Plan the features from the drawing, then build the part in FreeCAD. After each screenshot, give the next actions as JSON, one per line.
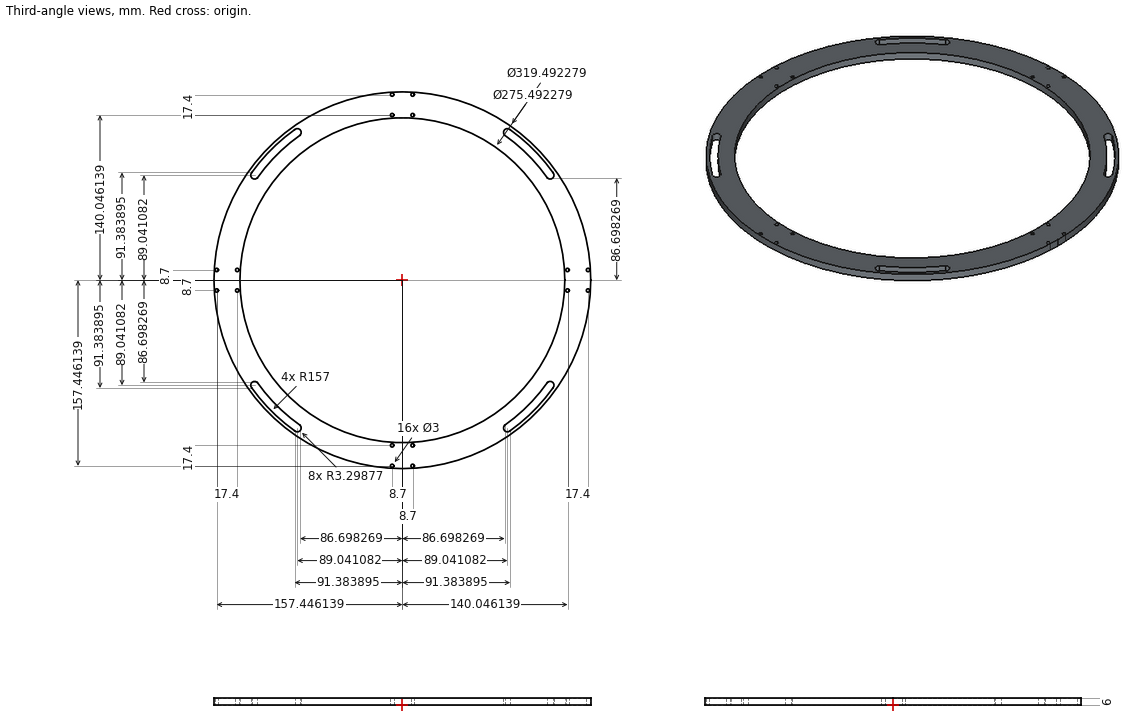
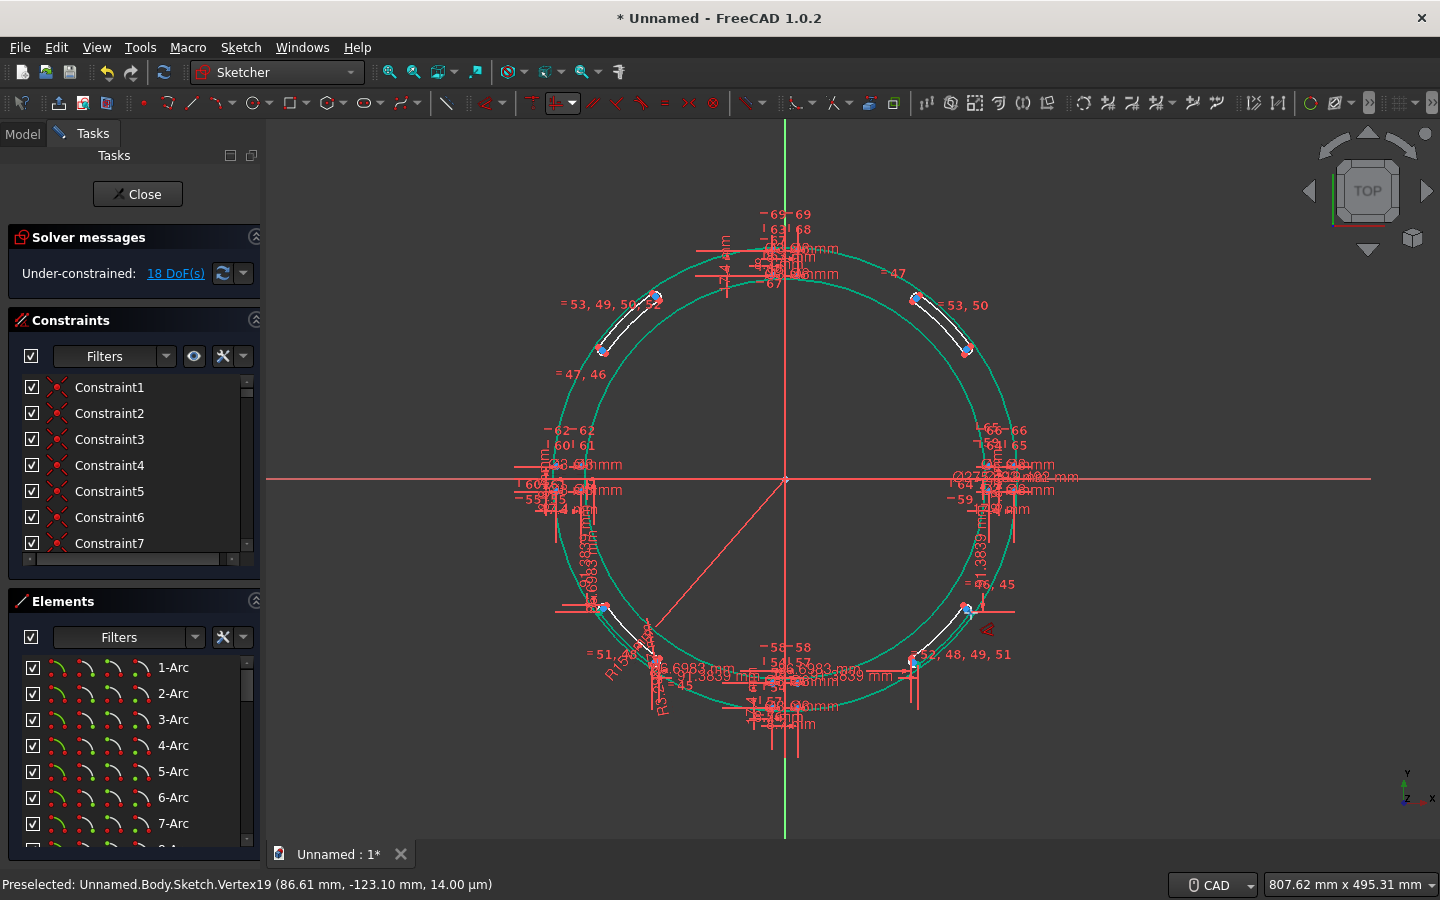
{"action": "scroll", "coordinate": [599, 347], "scroll_direction": "up", "scroll_amount": 5}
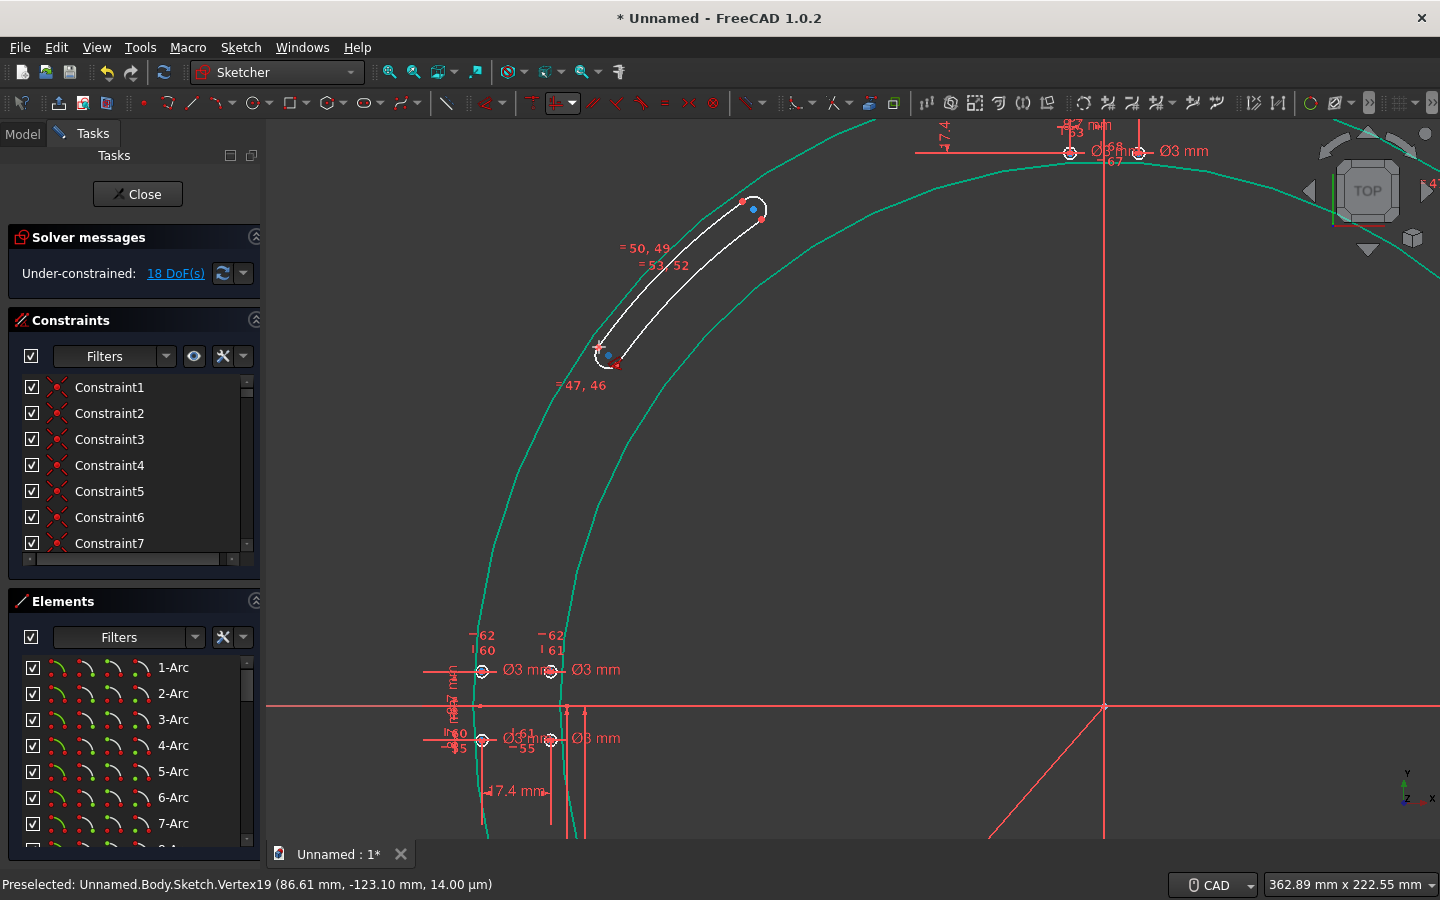
{"action": "left_click", "coordinate": [598, 348]}
{"action": "left_click", "coordinate": [564, 527]}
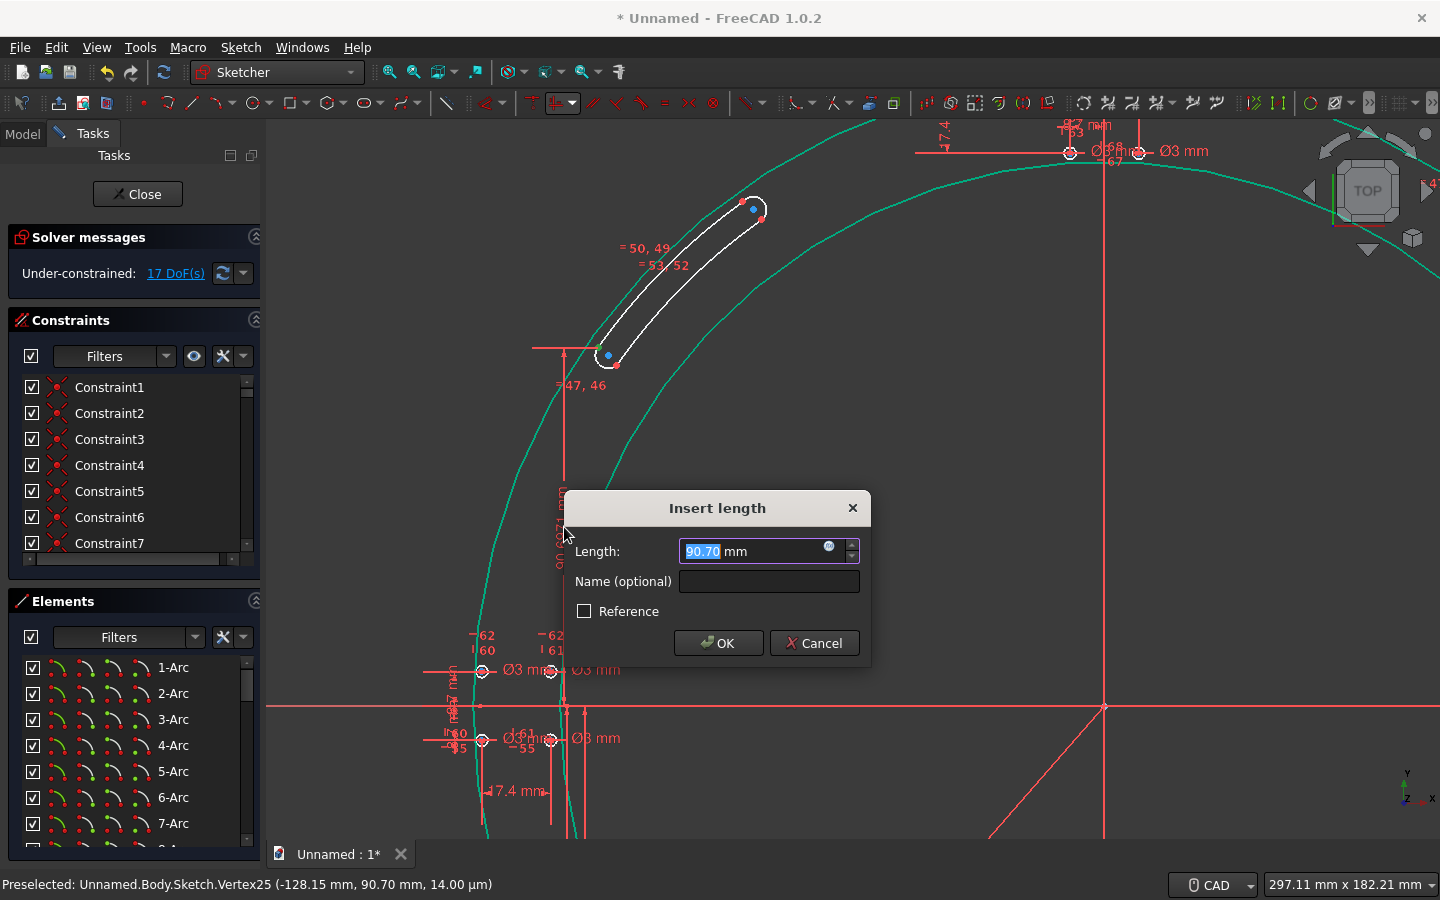
{"action": "type", "text": "91.383895"}
{"action": "key", "text": "Return"}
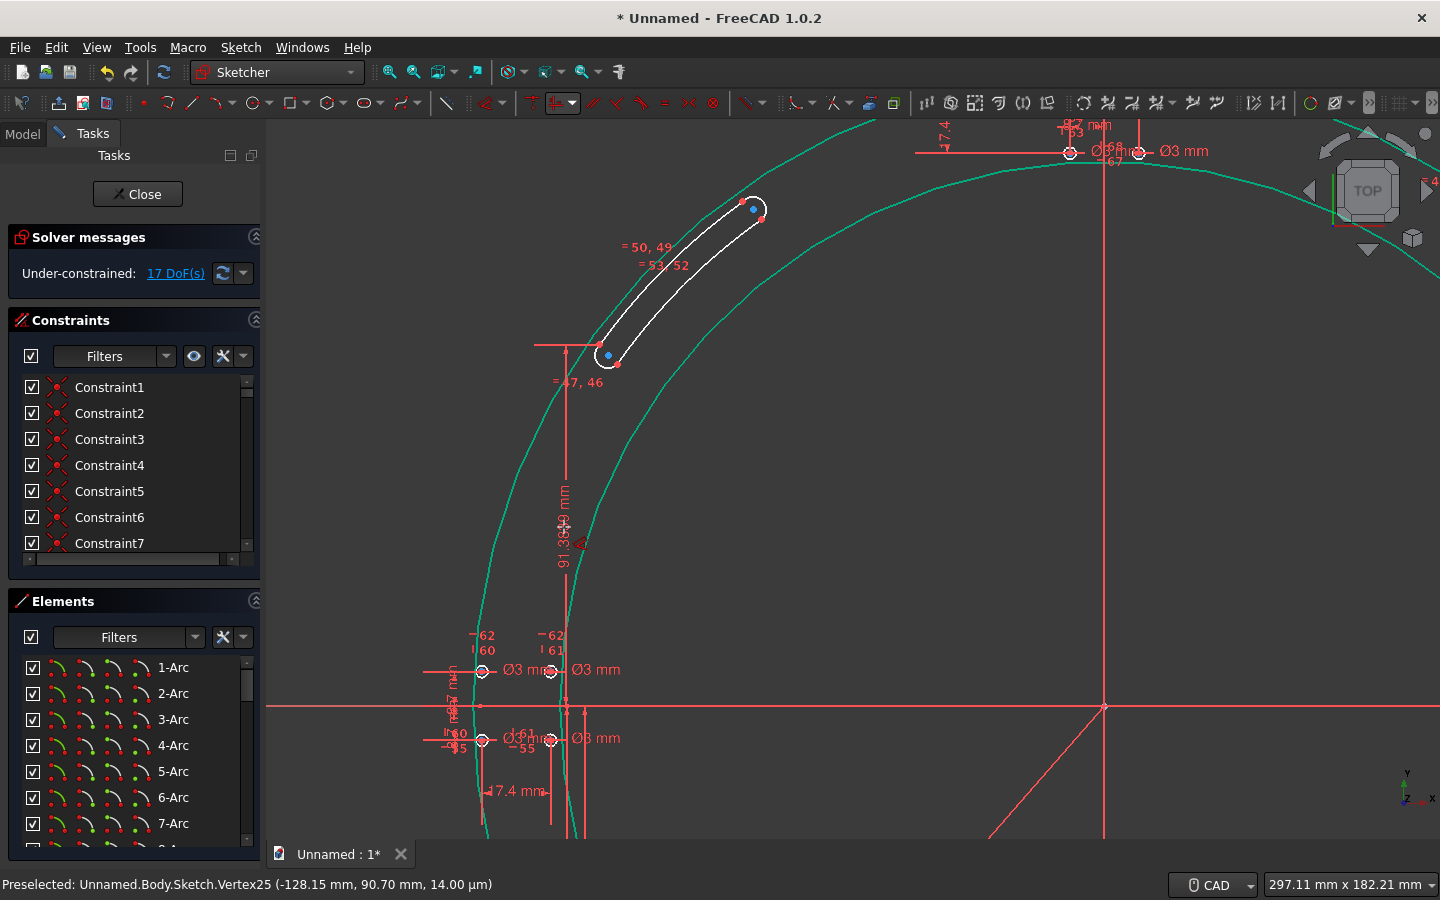
{"action": "left_click", "coordinate": [743, 202]}
{"action": "left_click", "coordinate": [924, 168]}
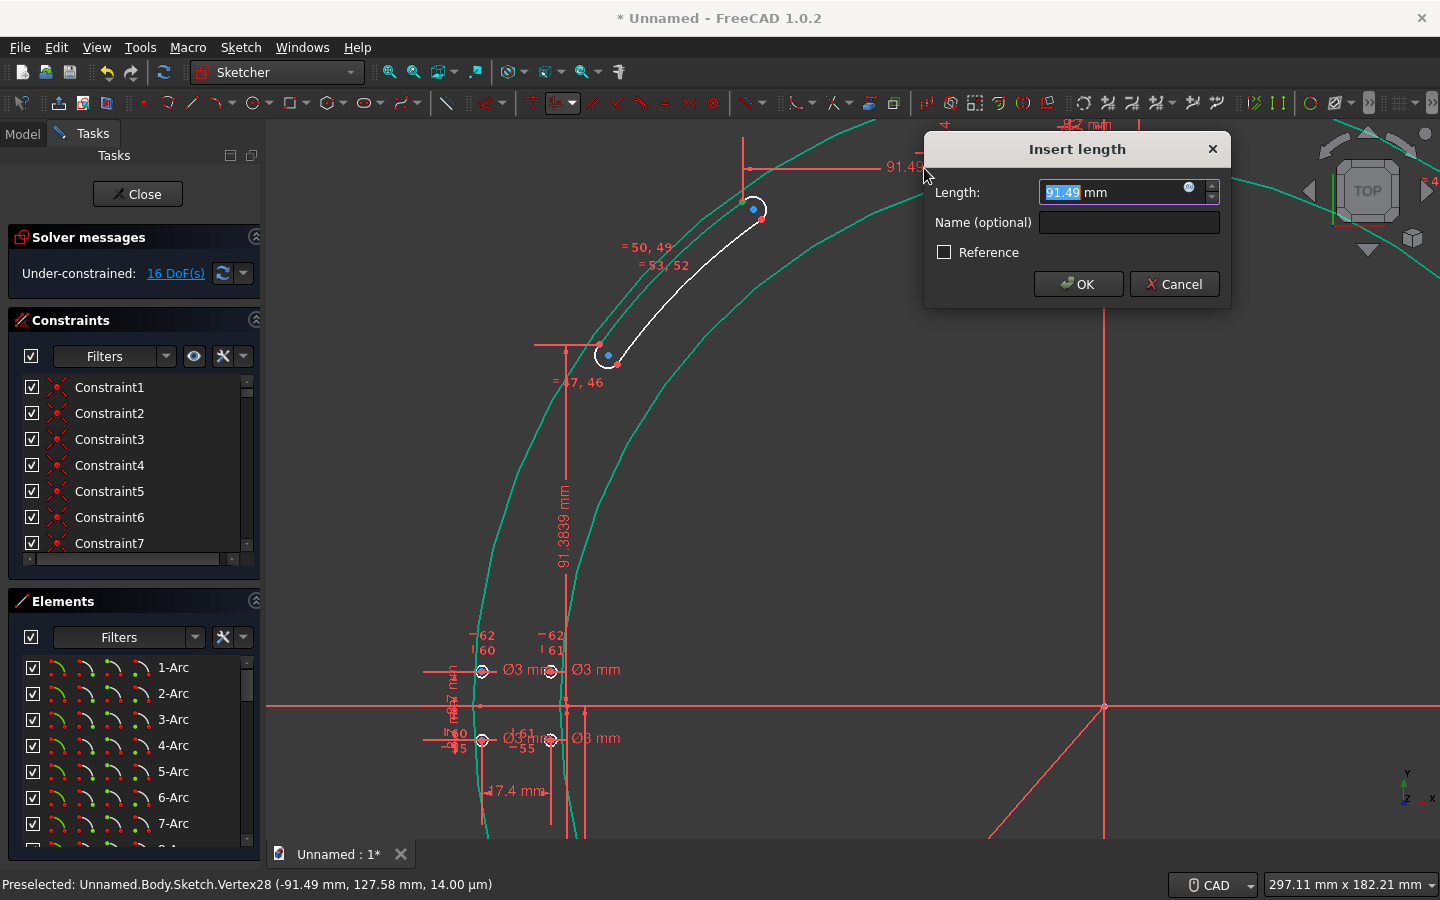
{"action": "type", "text": "91.383895"}
{"action": "key", "text": "Return"}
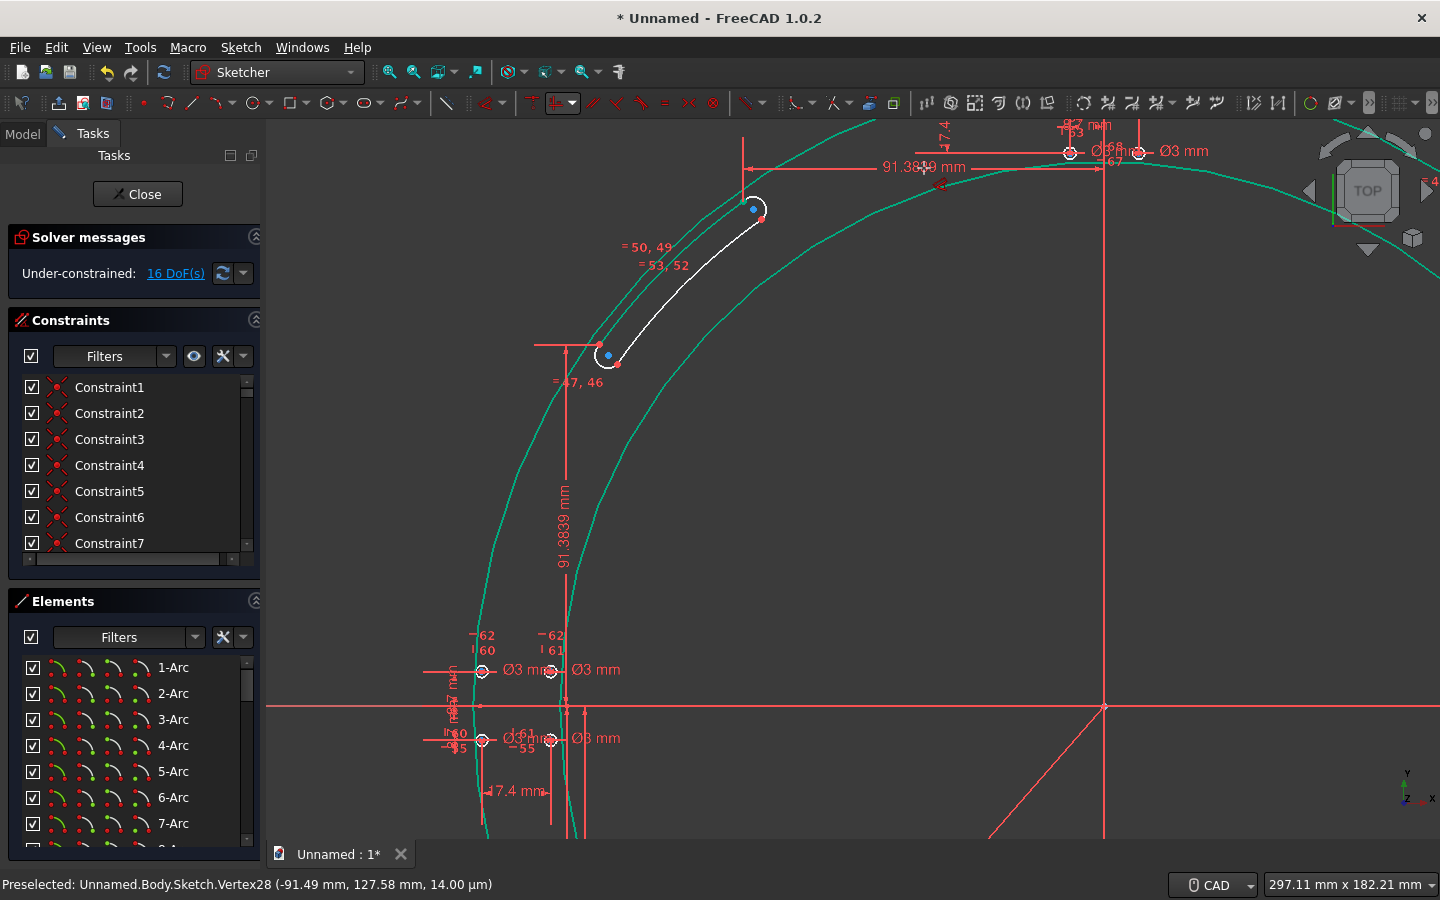
{"action": "left_click", "coordinate": [762, 219]}
{"action": "left_click", "coordinate": [1012, 185]}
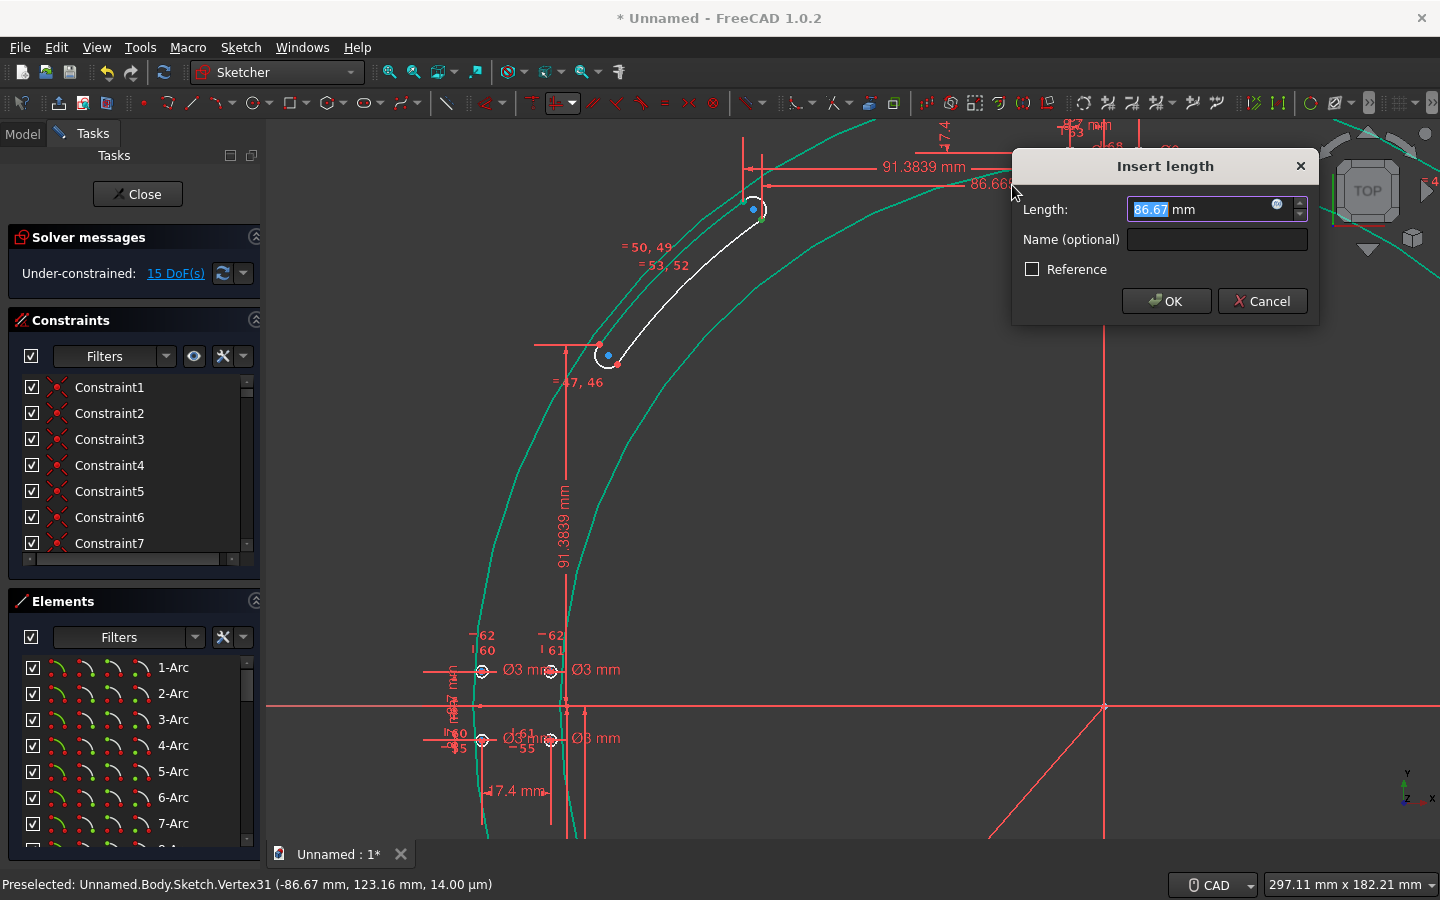
{"action": "type", "text": "86.698269"}
{"action": "key", "text": "Return"}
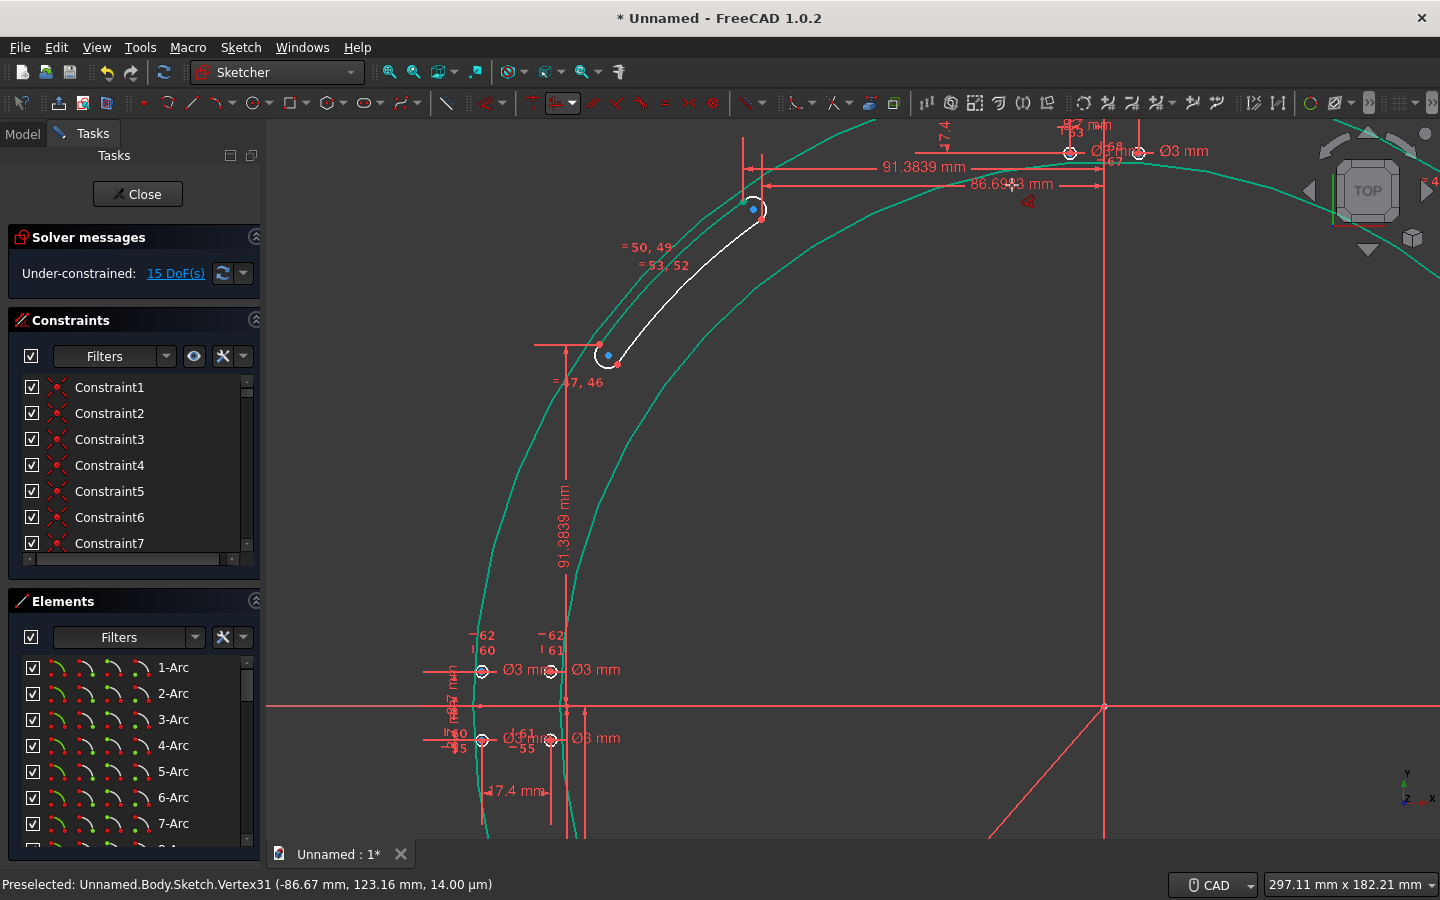
{"action": "scroll", "coordinate": [598, 347], "scroll_direction": "down", "scroll_amount": 5}